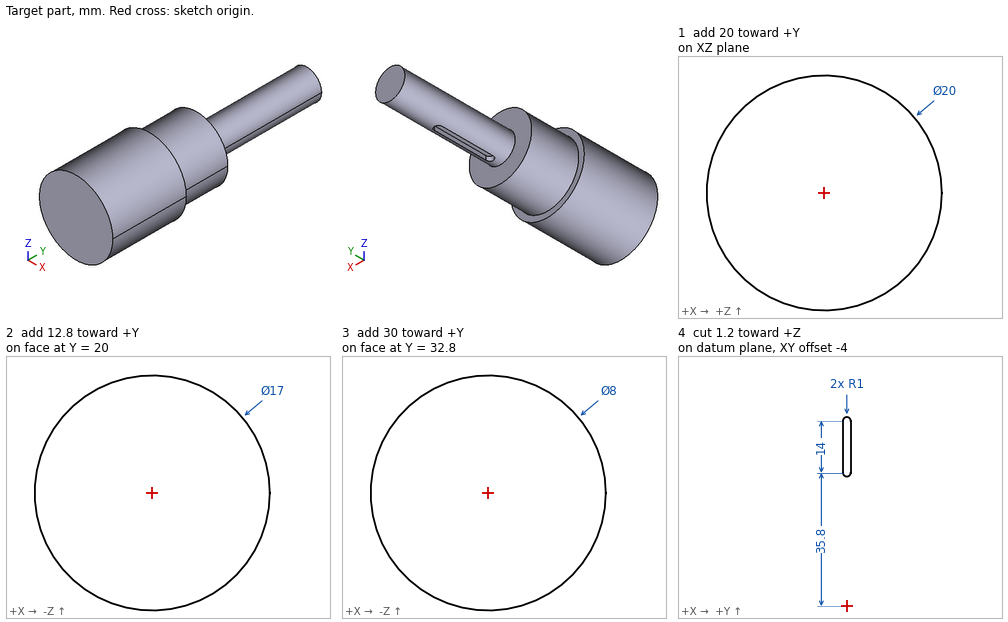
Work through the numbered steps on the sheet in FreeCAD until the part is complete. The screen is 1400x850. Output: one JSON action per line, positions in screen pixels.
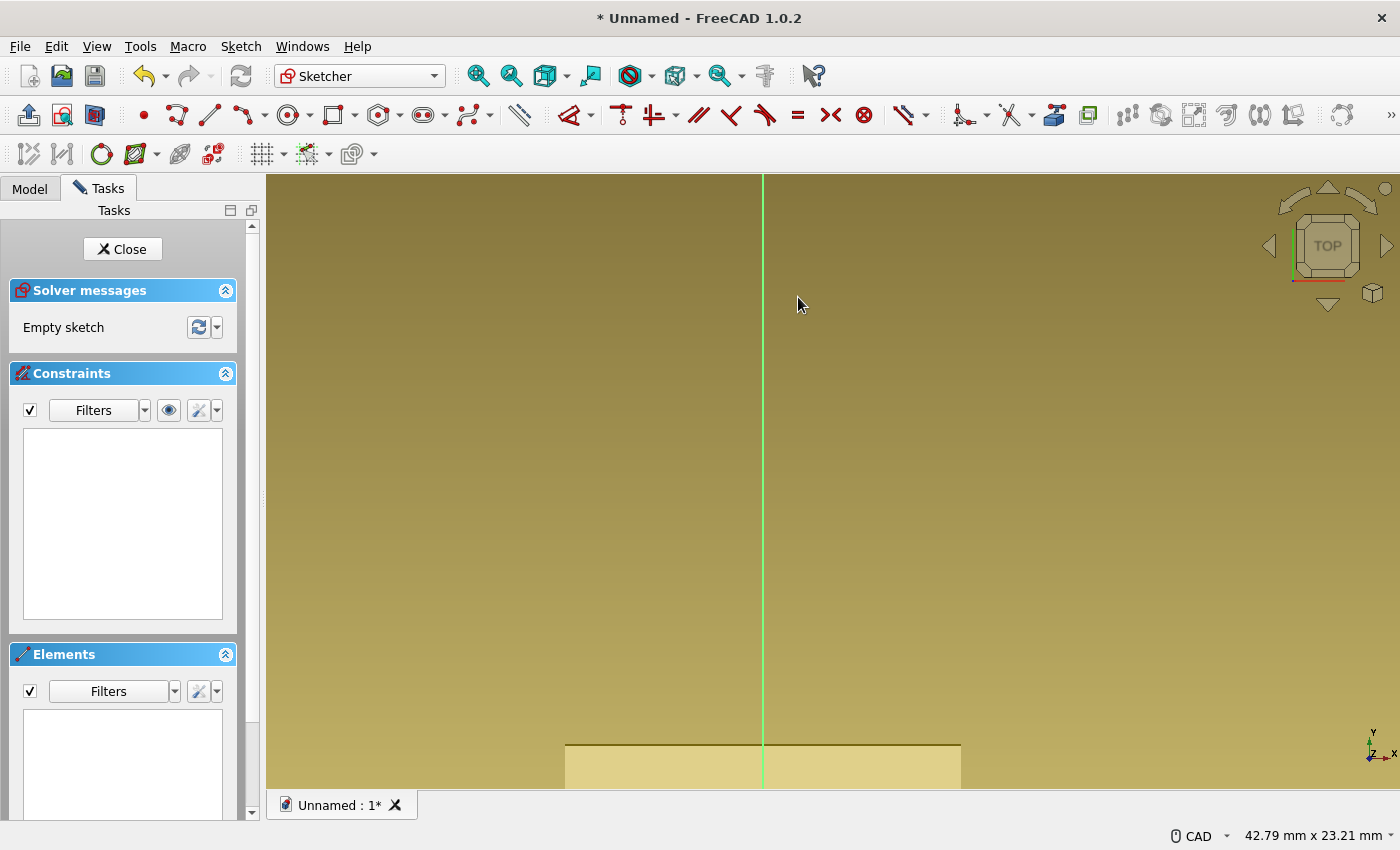
{"action": "left_click", "coordinate": [422, 116]}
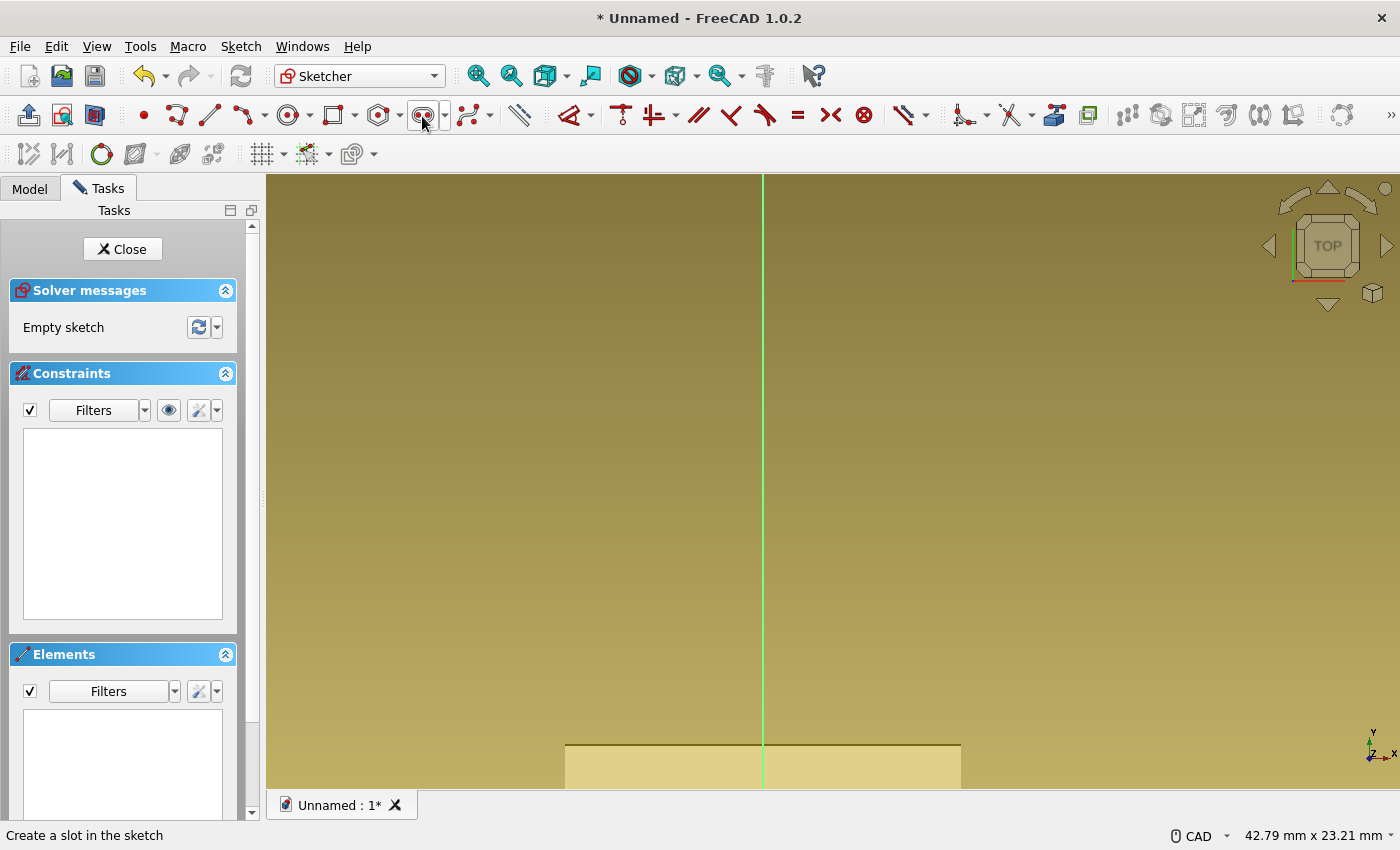
{"action": "left_click", "coordinate": [763, 666]}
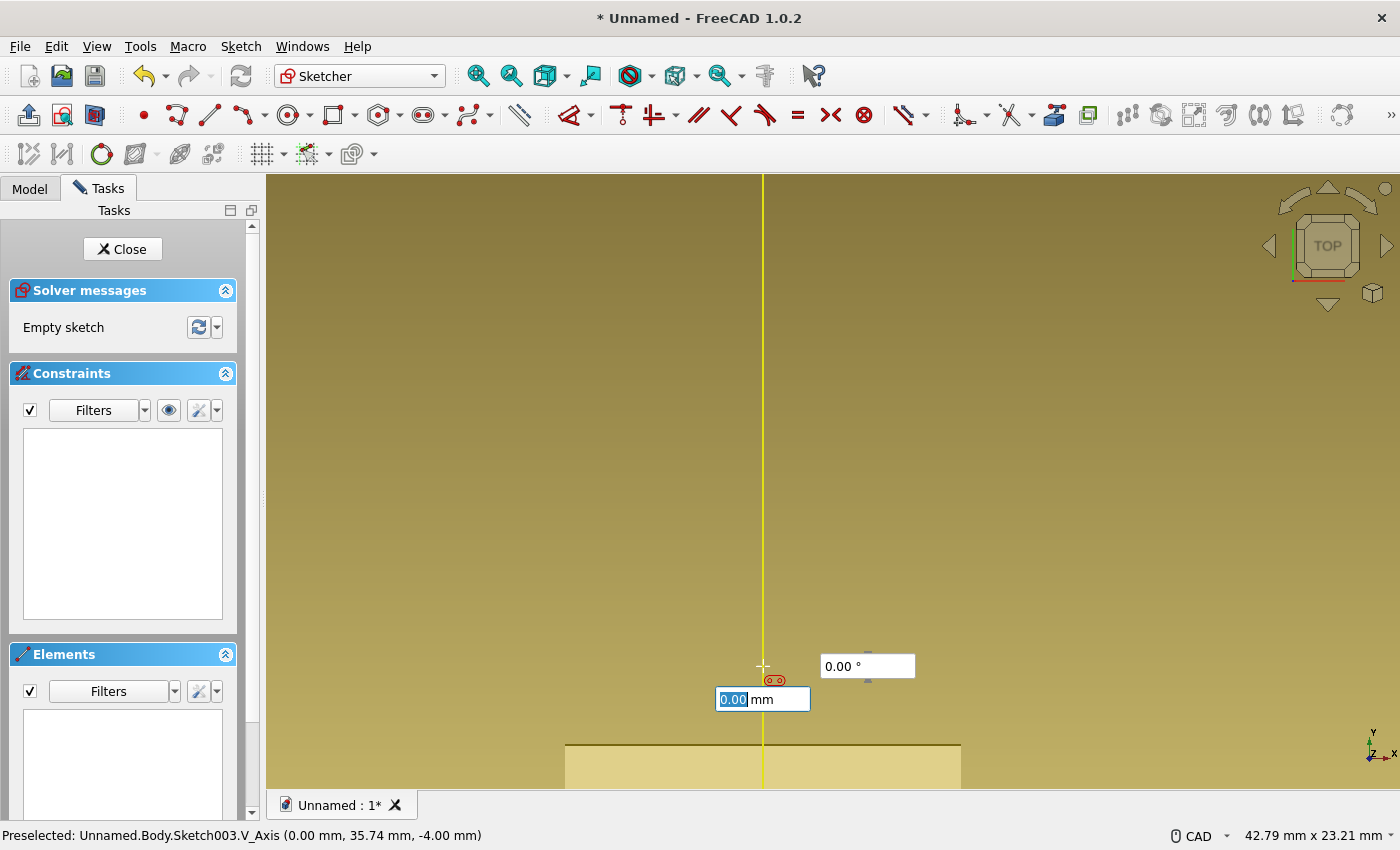
{"action": "left_click", "coordinate": [772, 294]}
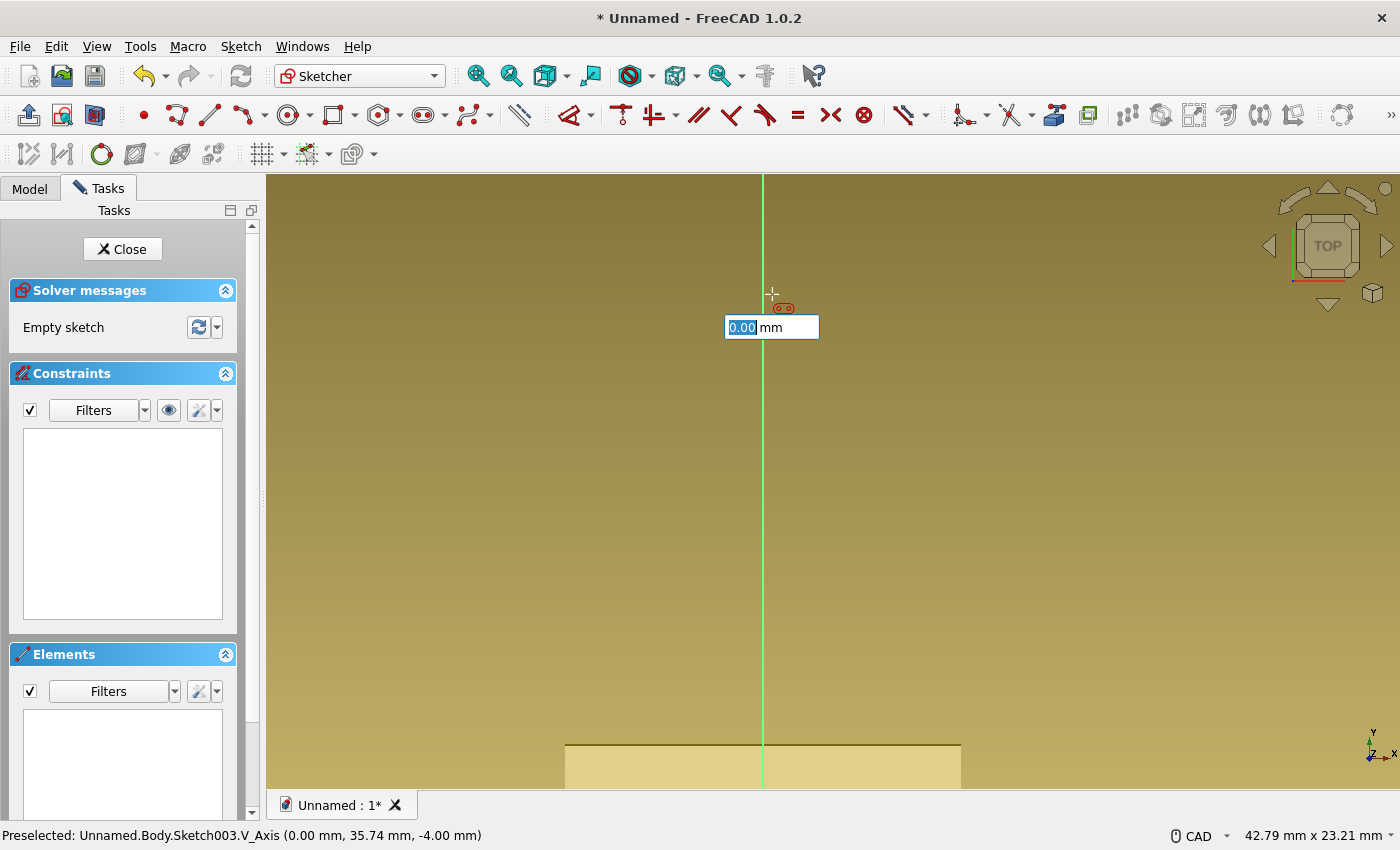
{"action": "left_click", "coordinate": [737, 480]}
{"action": "key", "text": "Escape"}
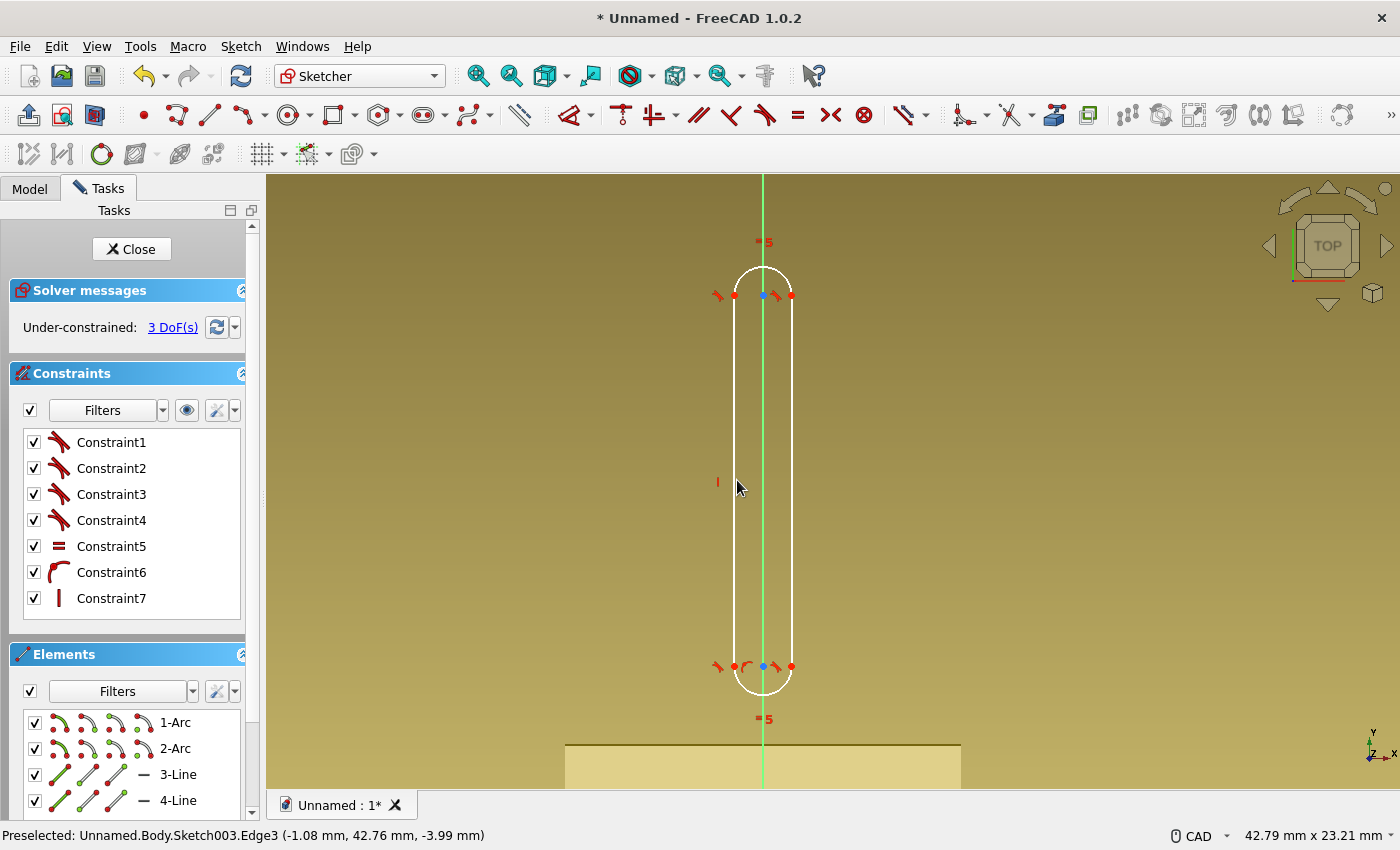
{"action": "left_click", "coordinate": [568, 116]}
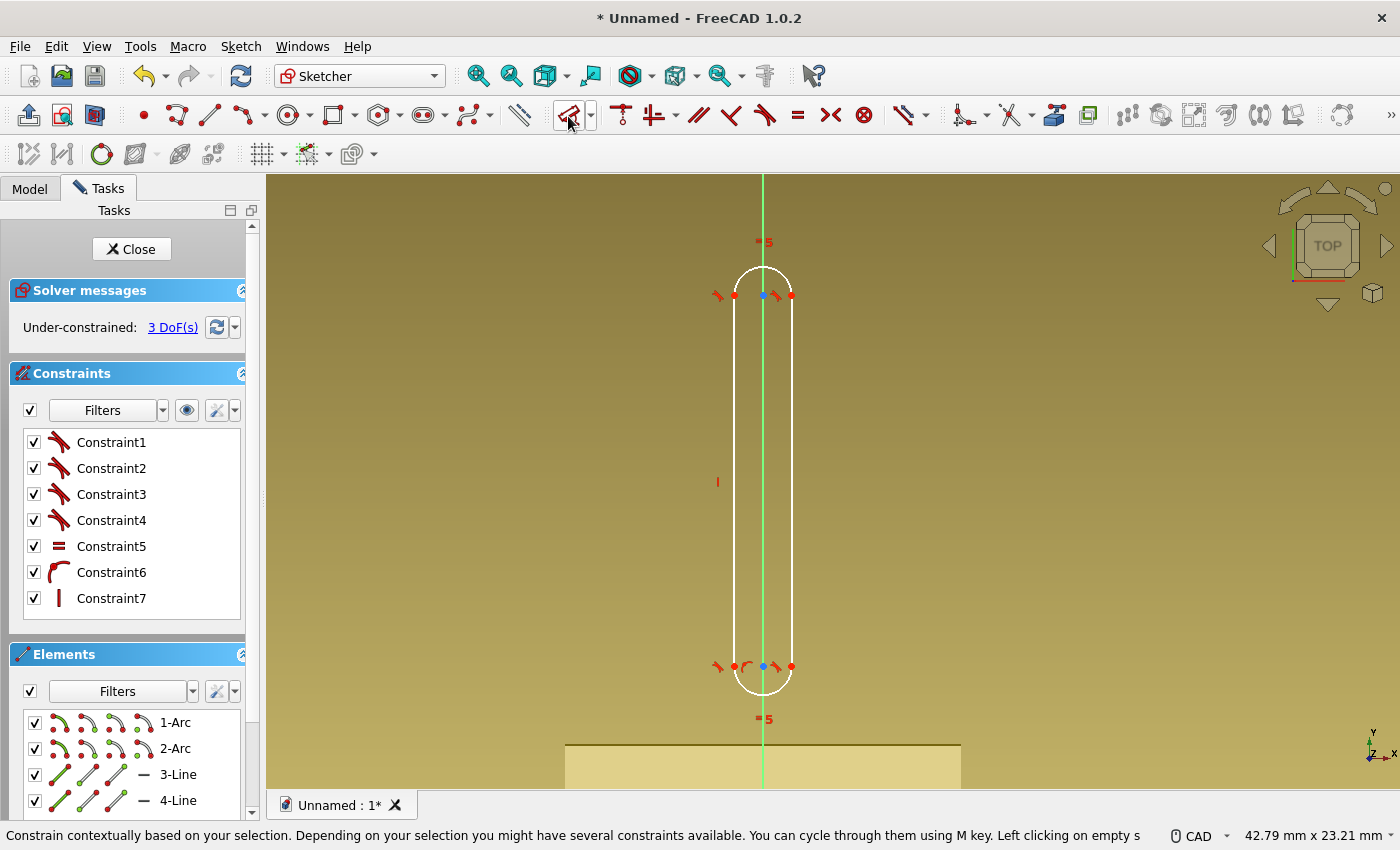
{"action": "scroll", "coordinate": [746, 690], "scroll_direction": "up", "scroll_amount": 3}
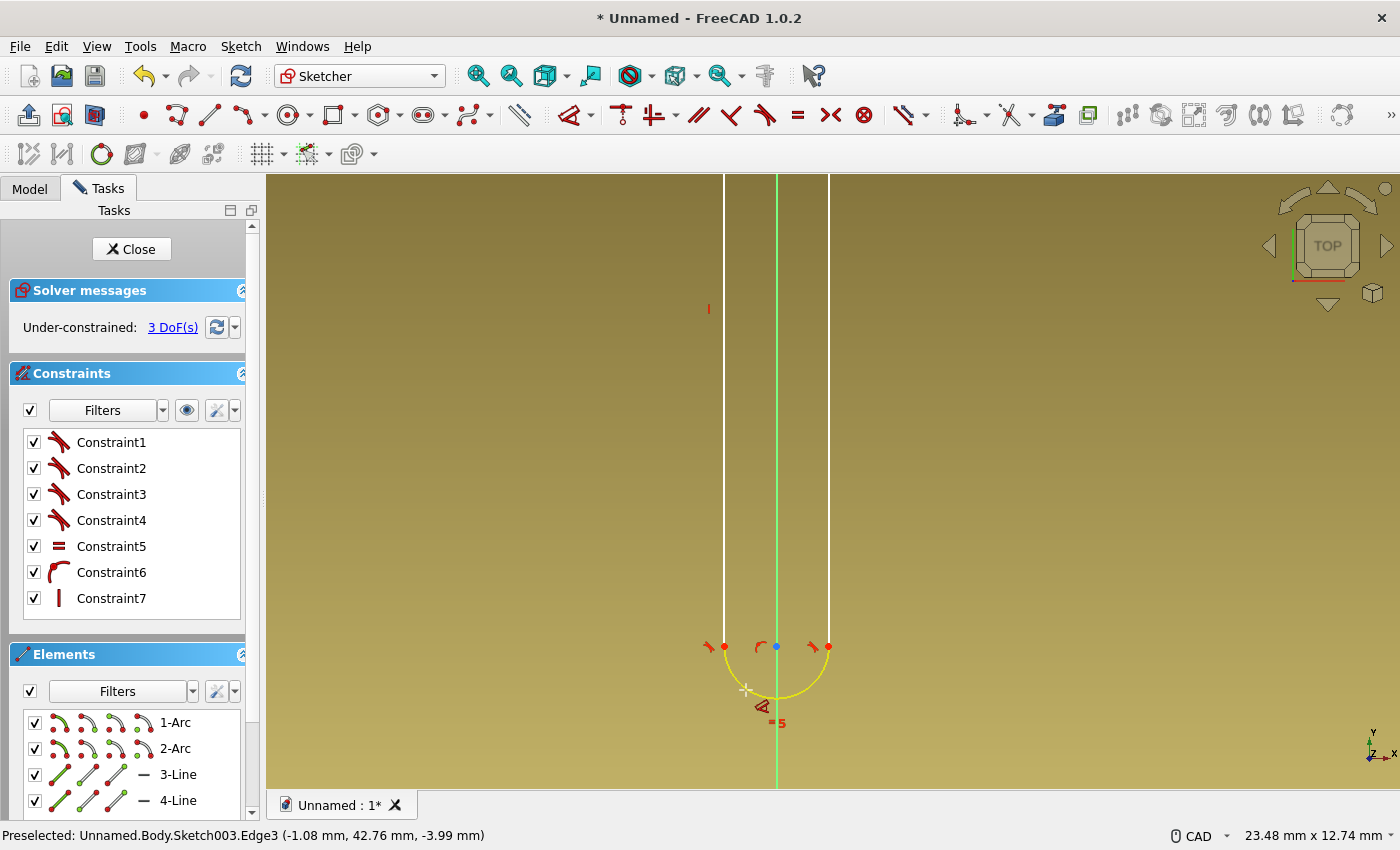
{"action": "left_click", "coordinate": [746, 689]}
{"action": "left_click", "coordinate": [727, 715]}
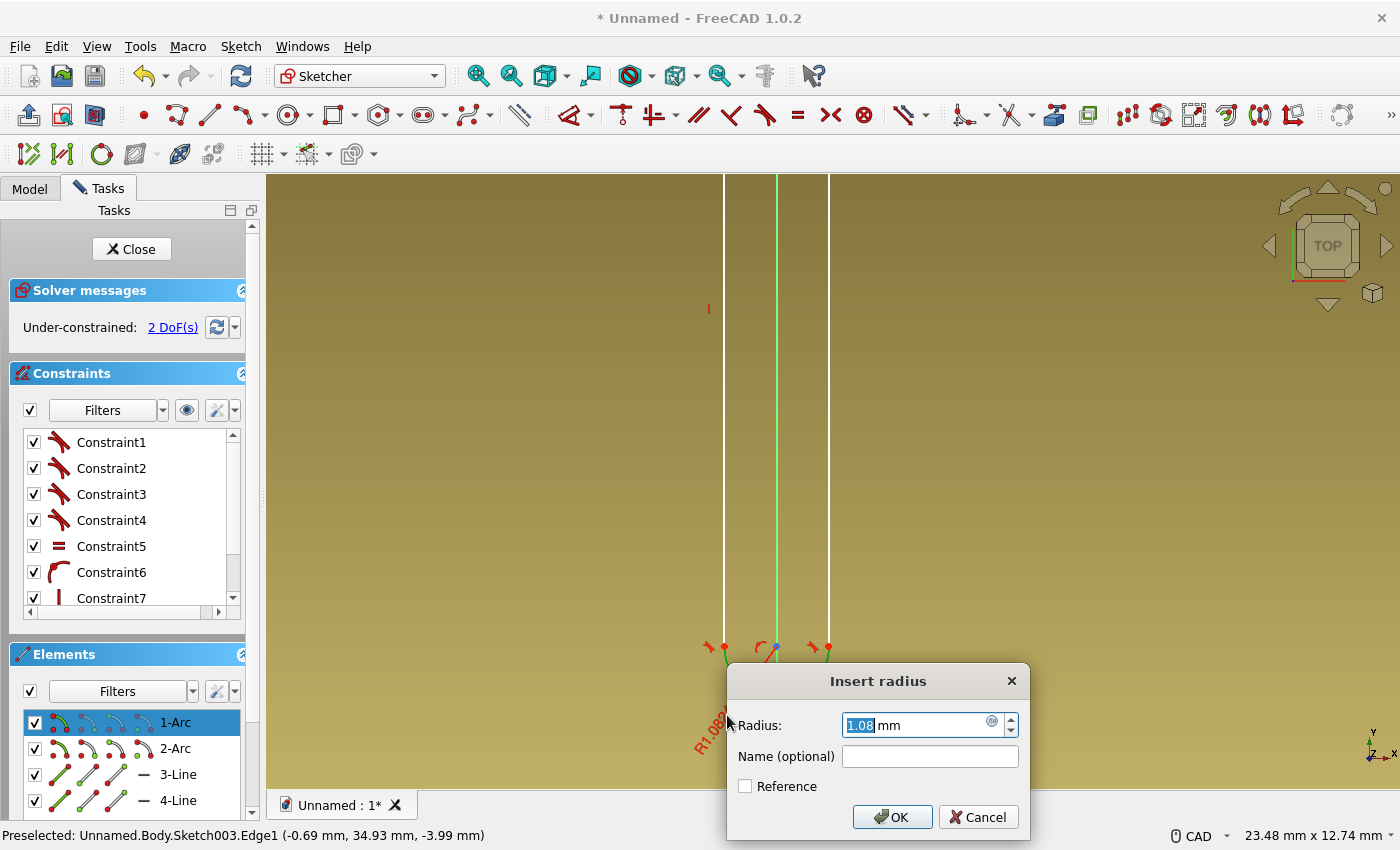
{"action": "type", "text": "1"}
{"action": "key", "text": "Return"}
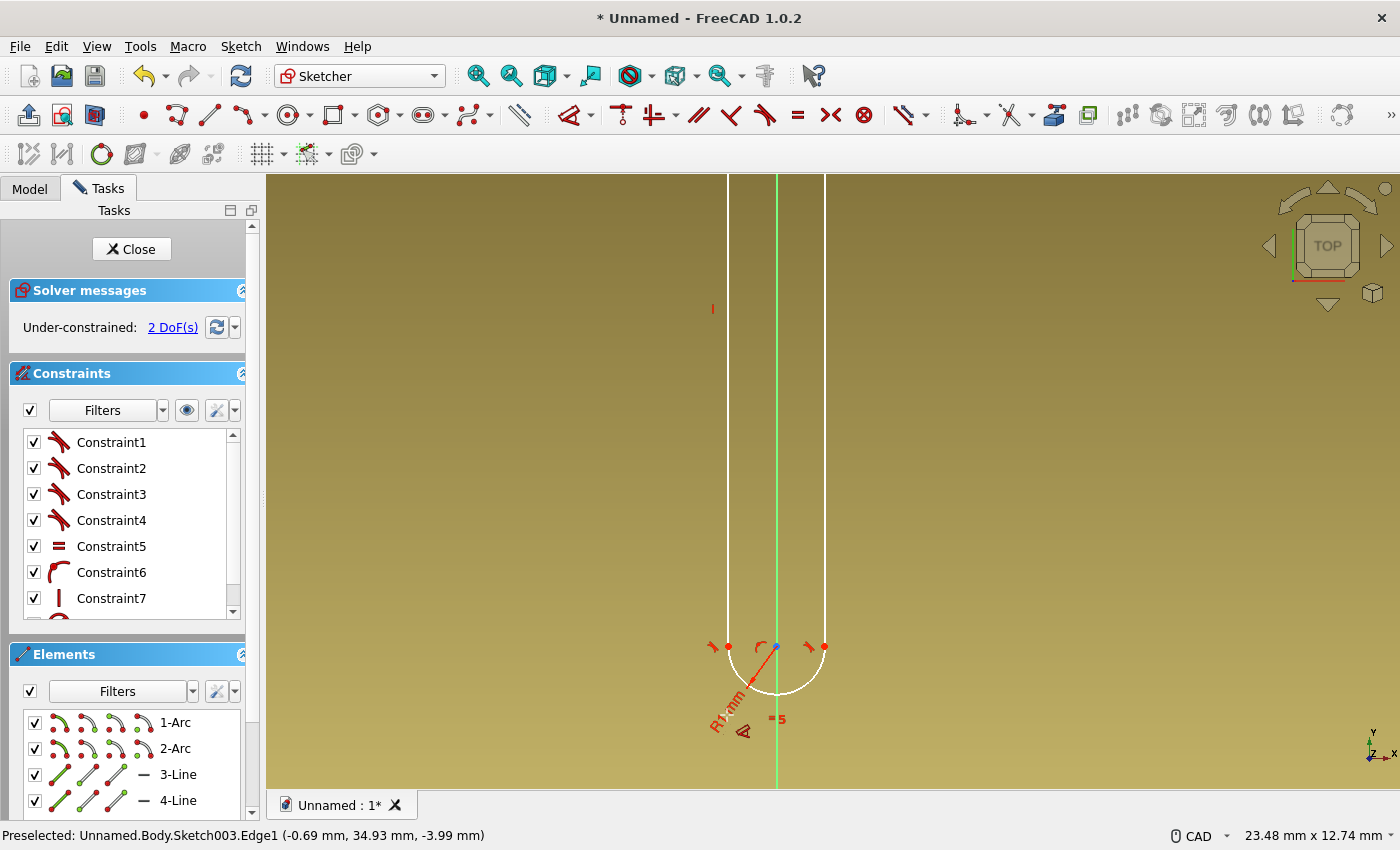
{"action": "left_click", "coordinate": [728, 444]}
{"action": "left_click", "coordinate": [694, 424]}